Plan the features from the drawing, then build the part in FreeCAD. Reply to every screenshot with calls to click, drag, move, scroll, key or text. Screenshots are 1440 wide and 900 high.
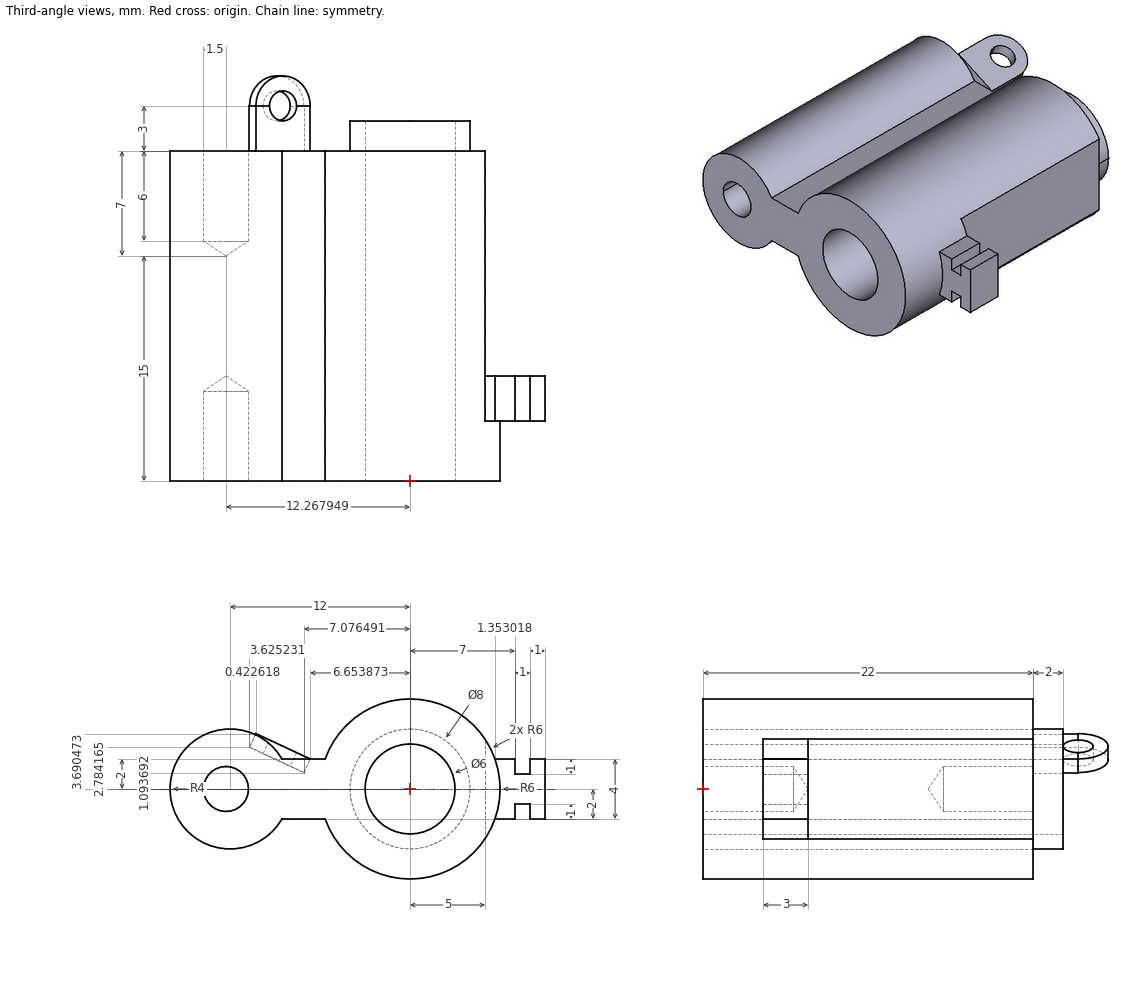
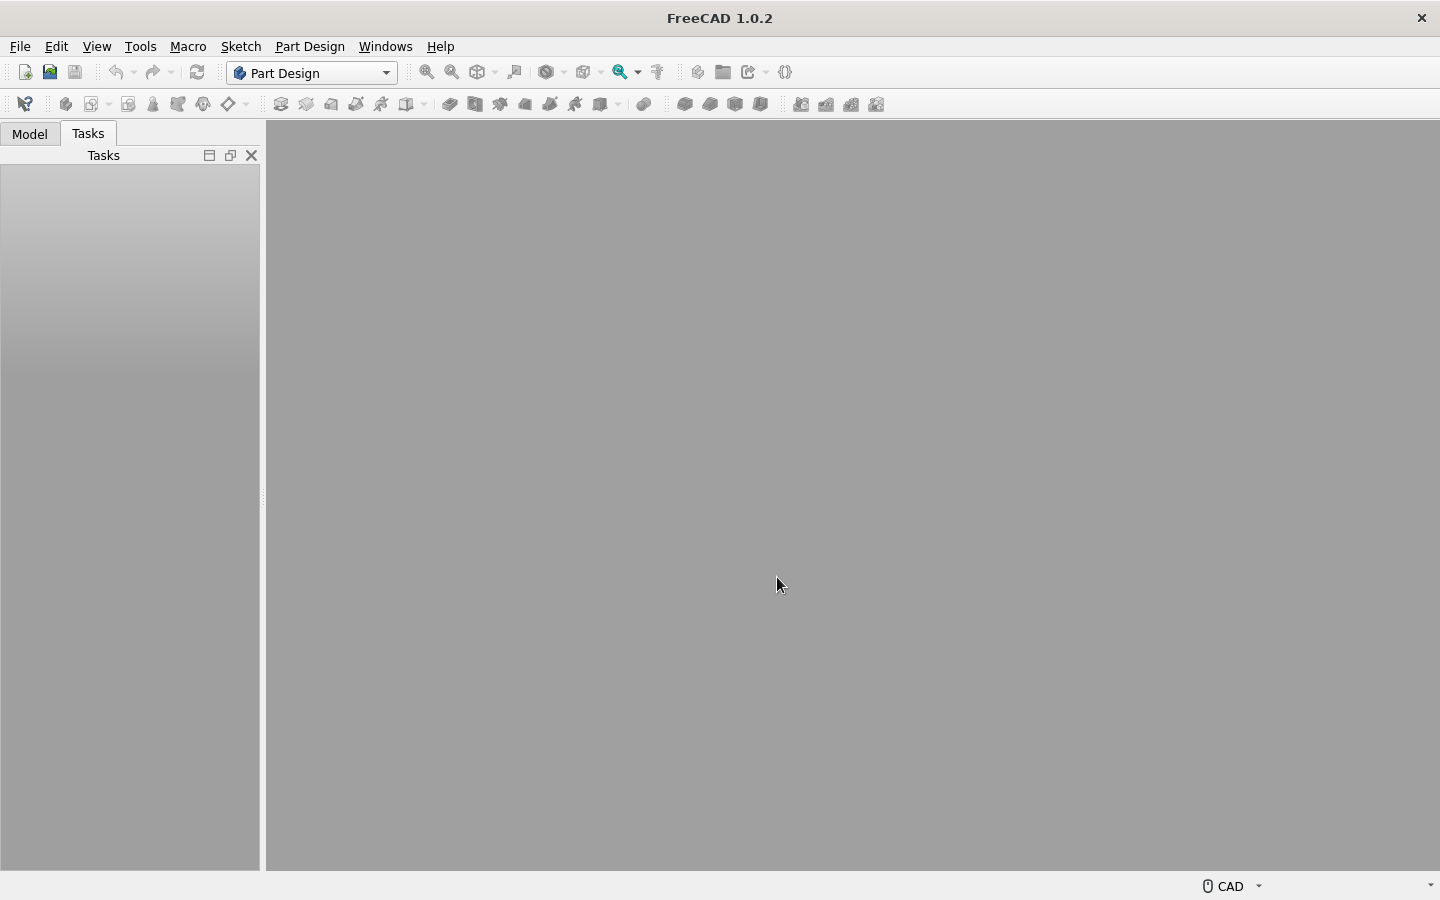
click(25, 72)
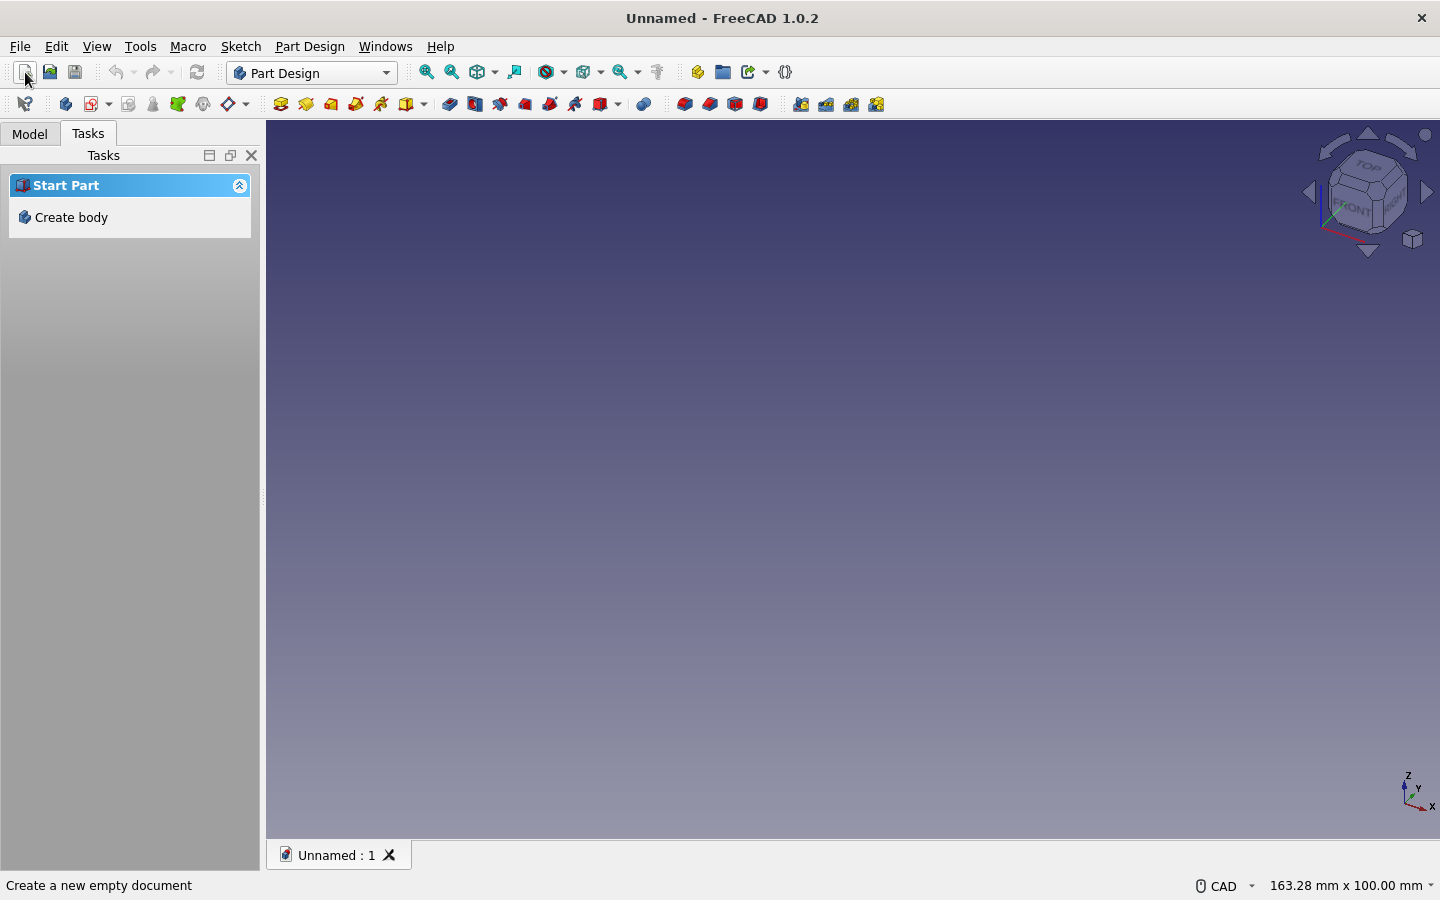
click(90, 104)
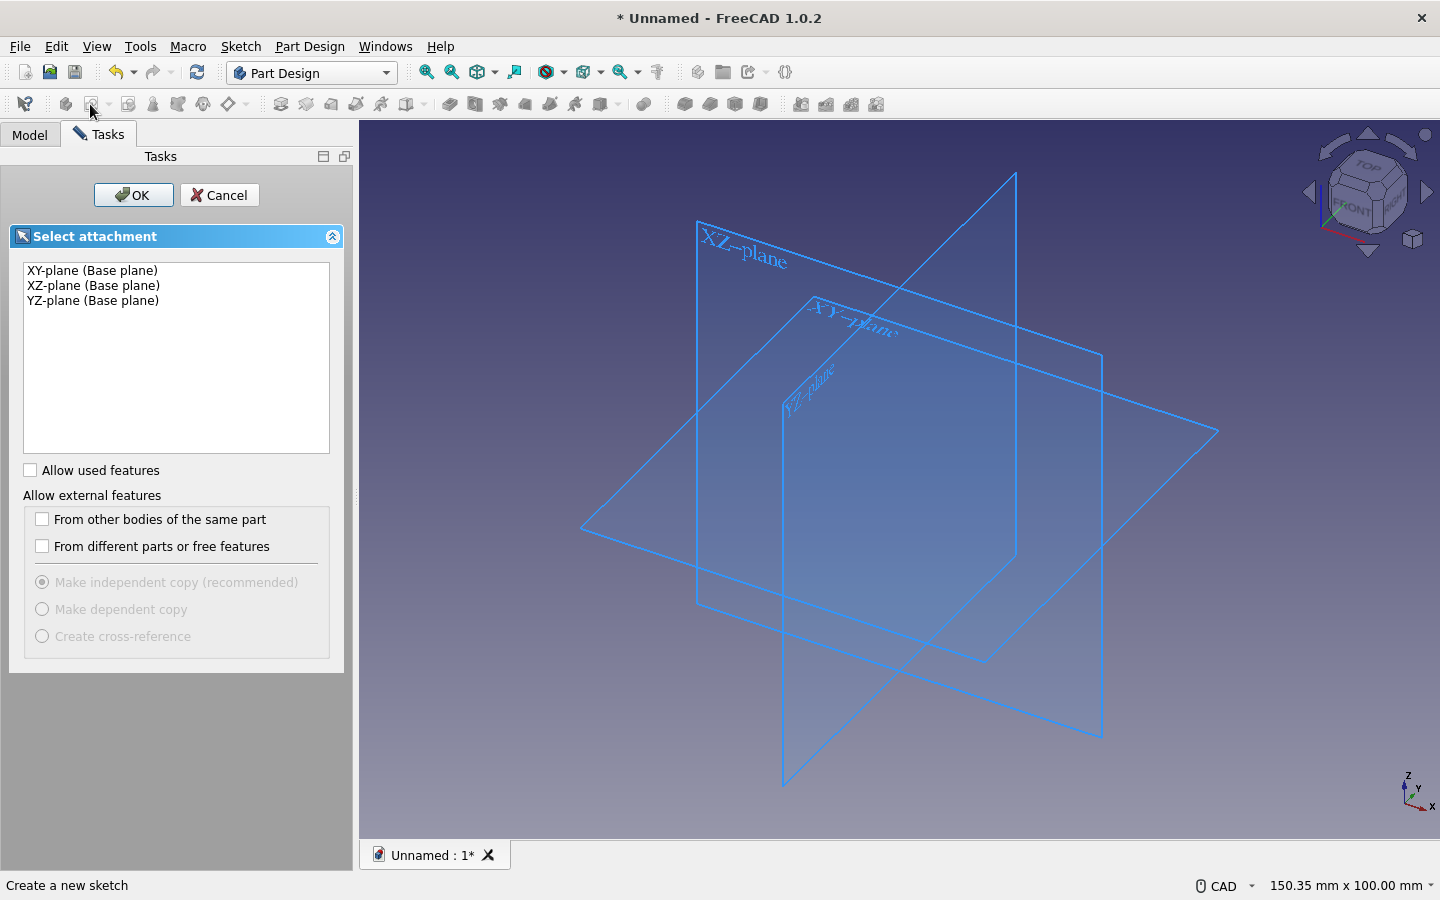
click(84, 286)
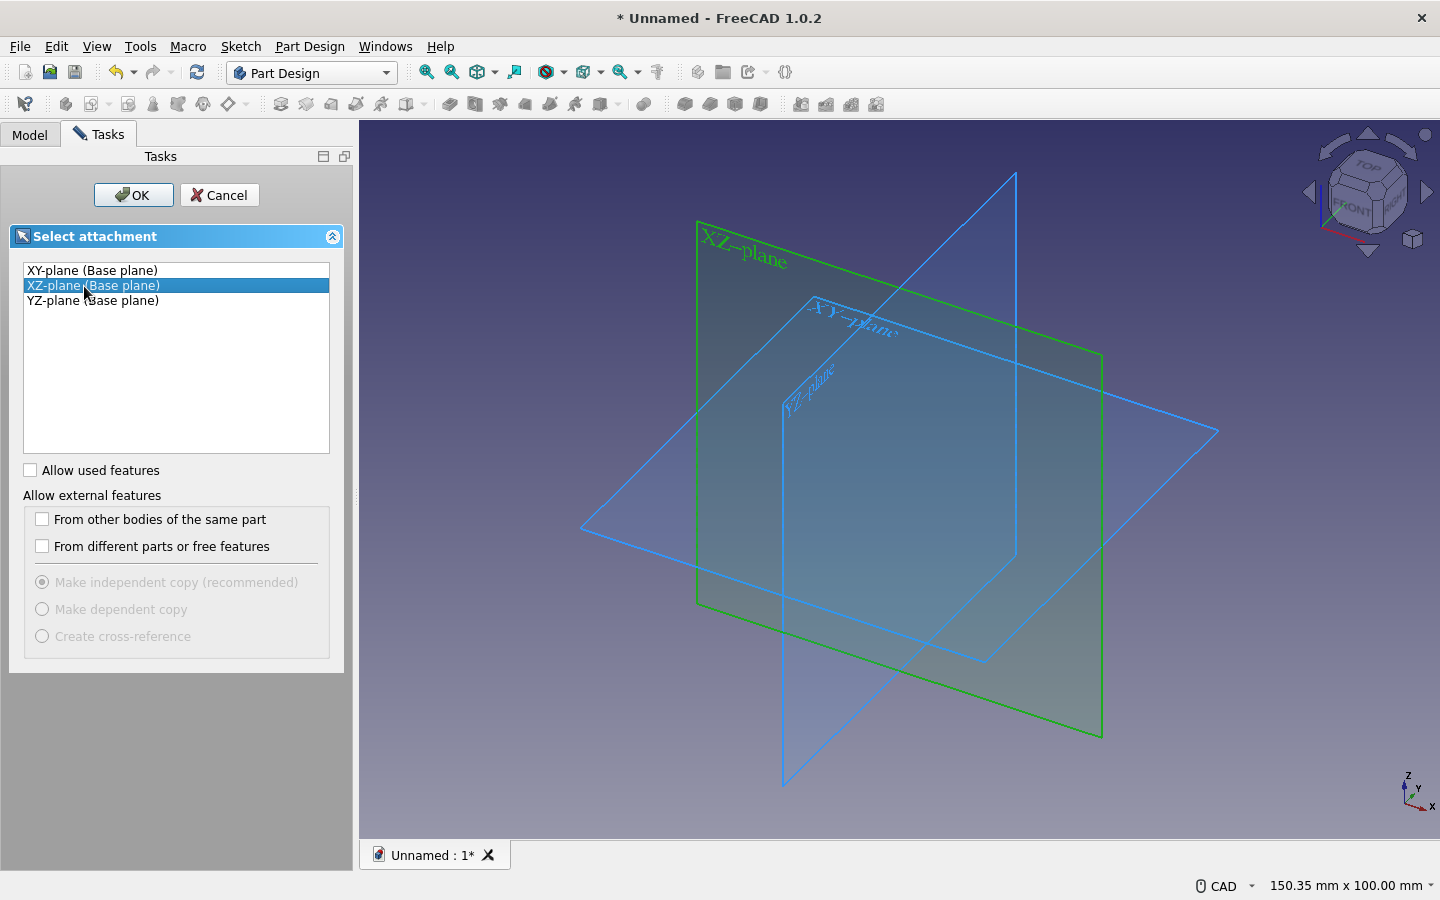
click(134, 195)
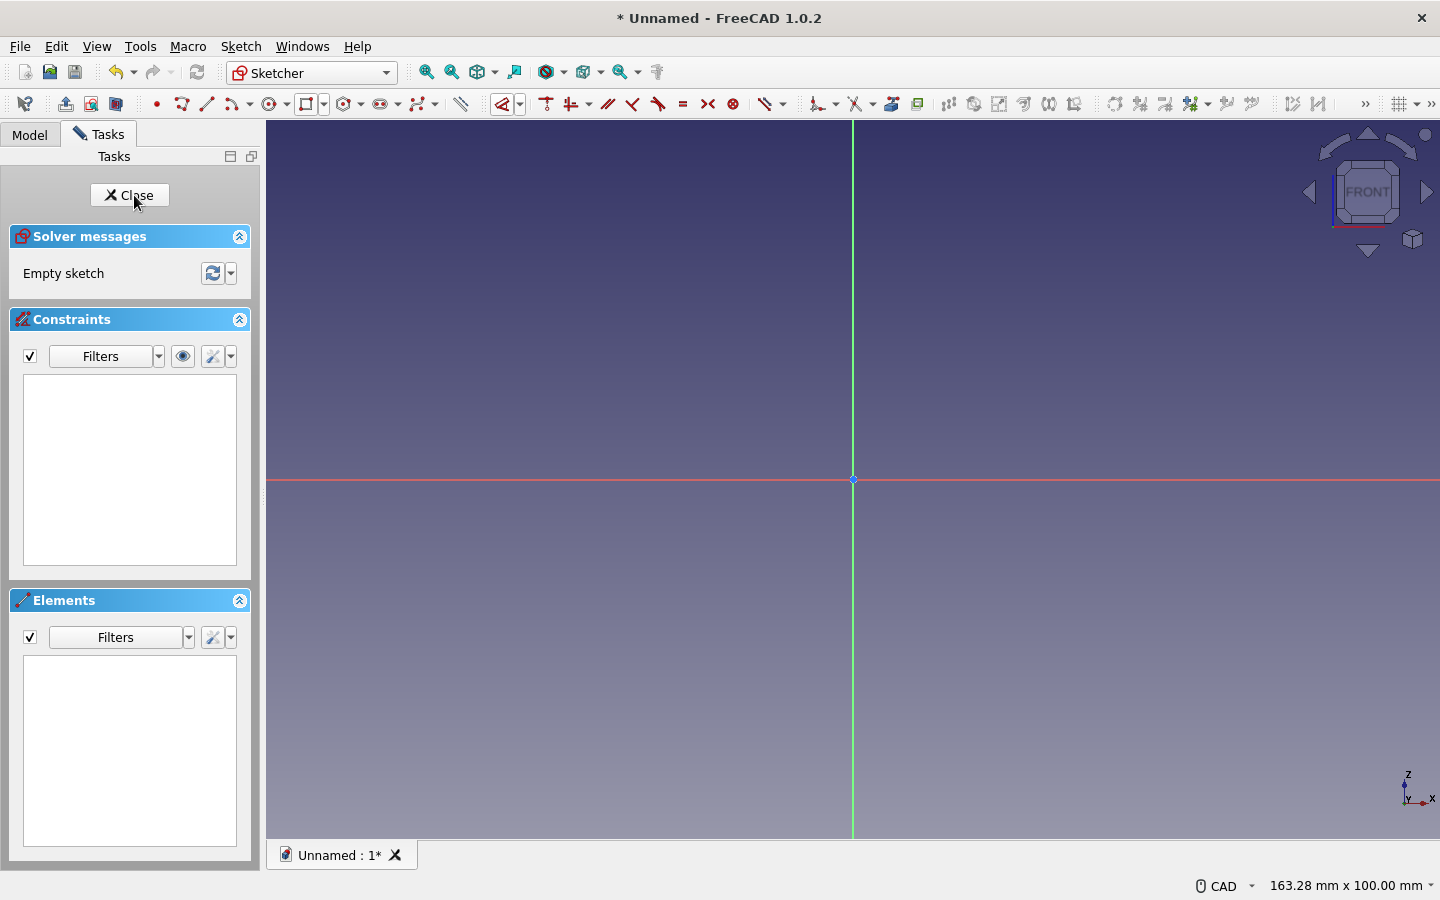
scroll(828, 480, up, 7)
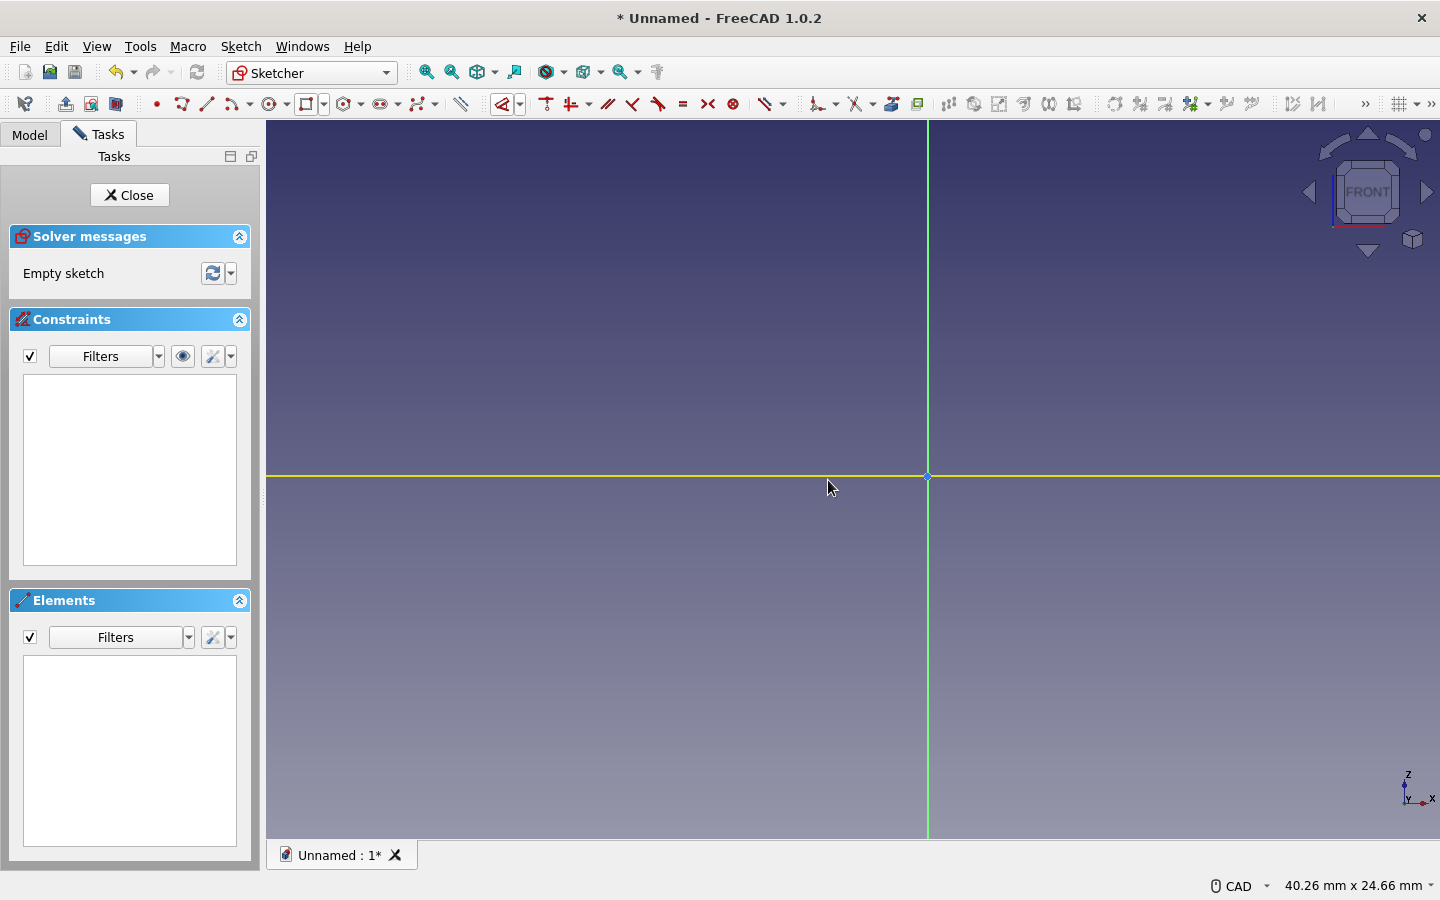
click(207, 104)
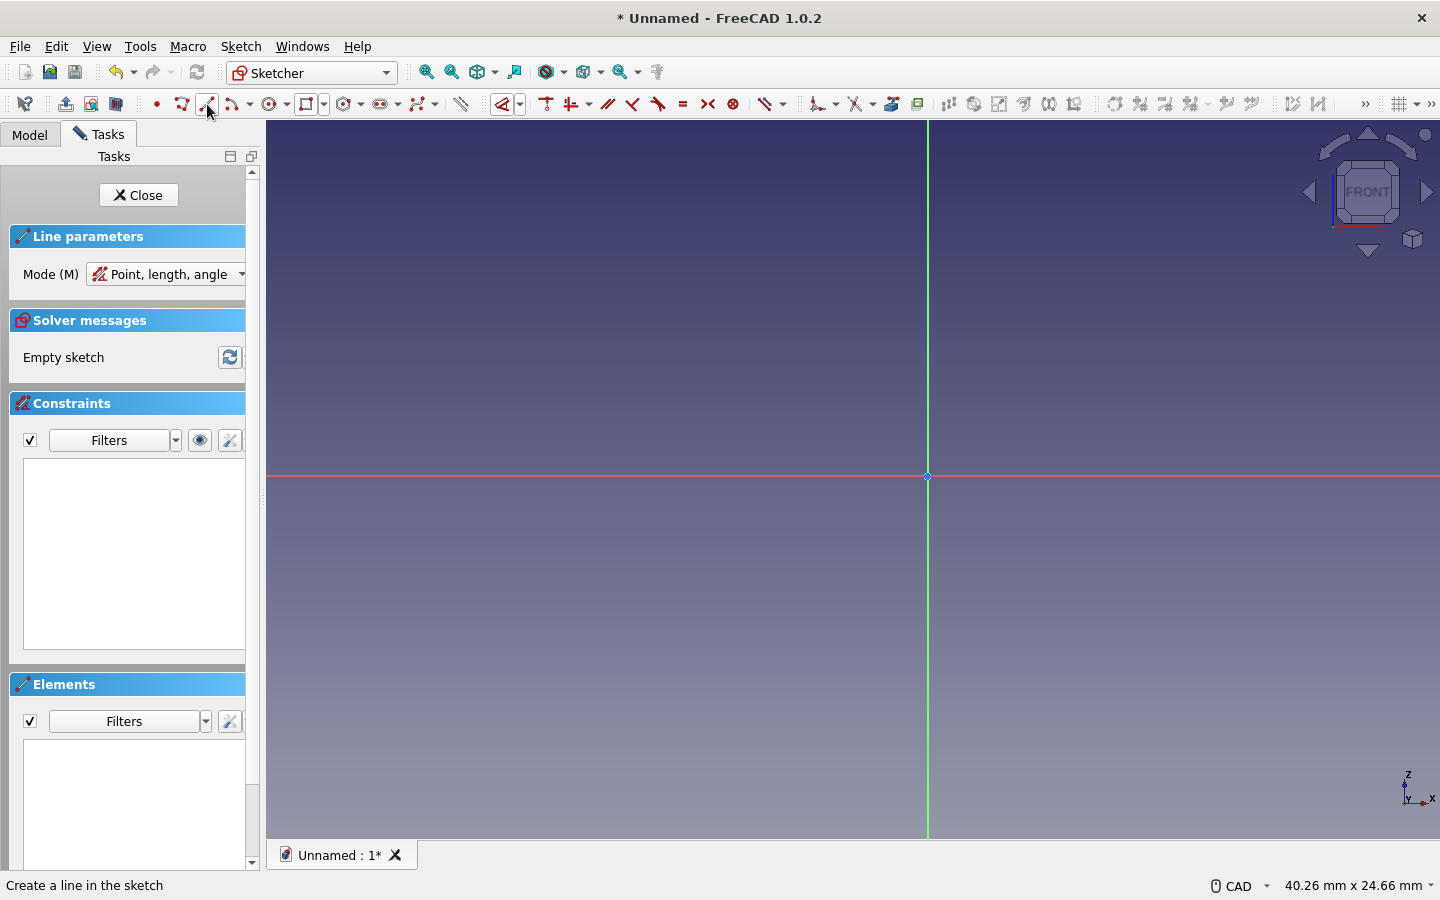
click(763, 535)
click(679, 535)